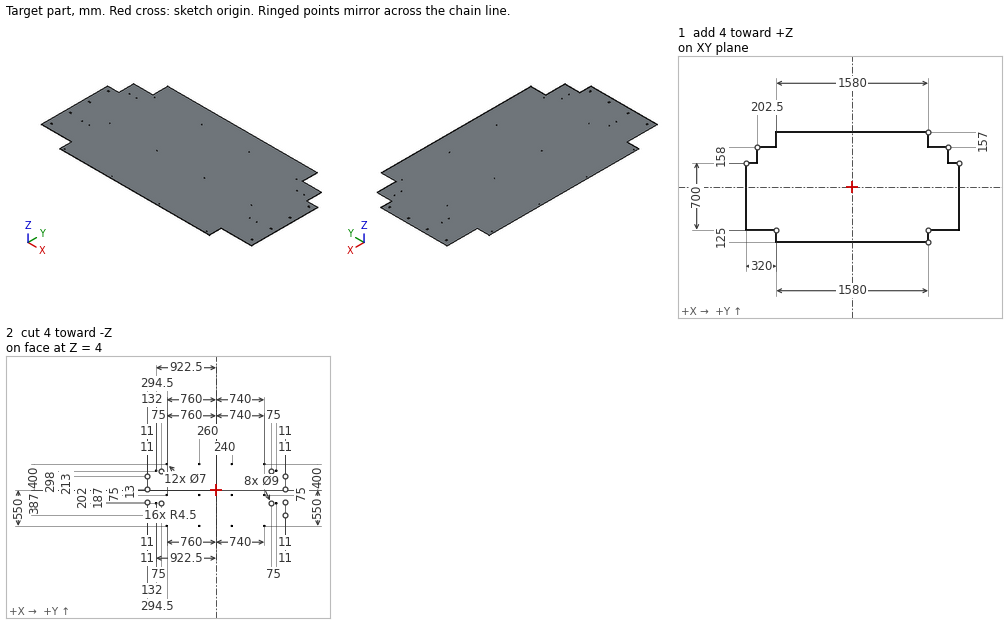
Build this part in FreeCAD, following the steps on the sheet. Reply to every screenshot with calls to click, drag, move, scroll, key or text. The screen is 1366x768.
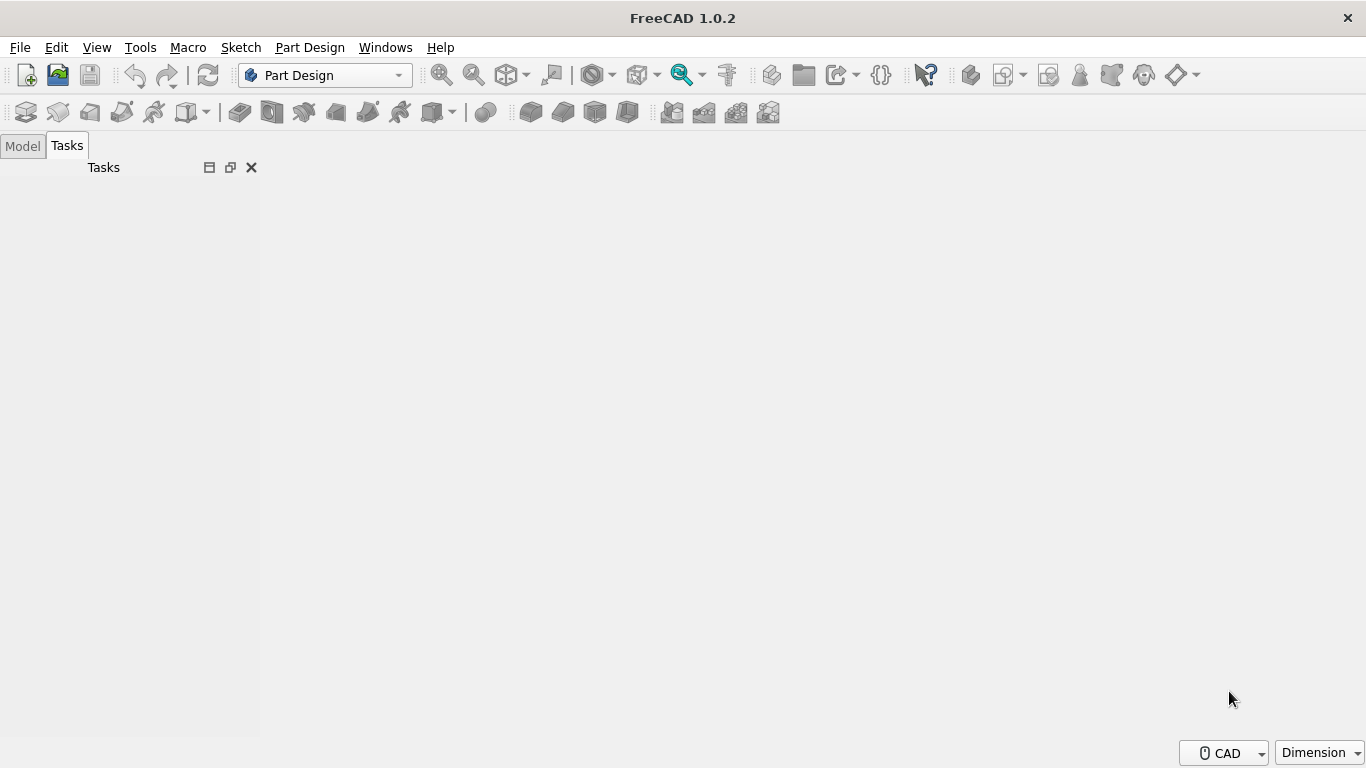
click(26, 76)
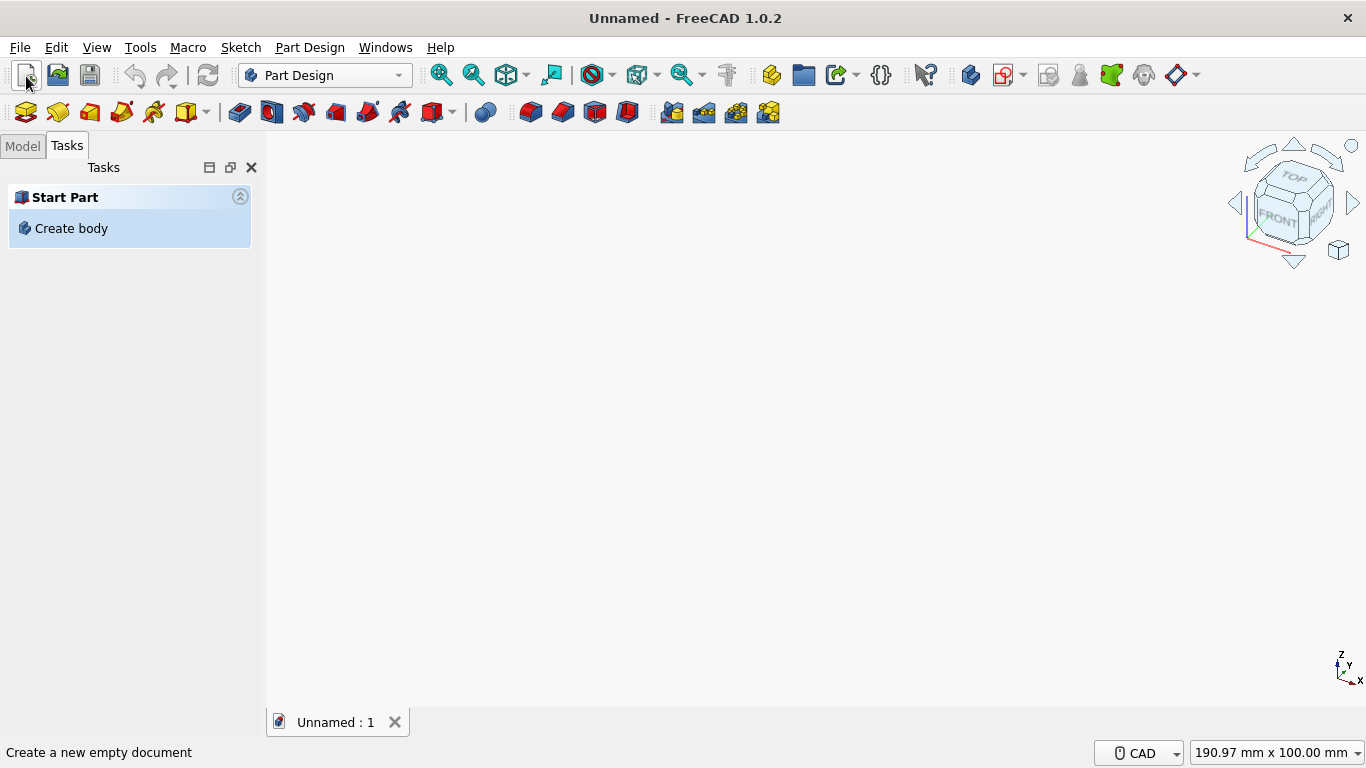
click(1004, 76)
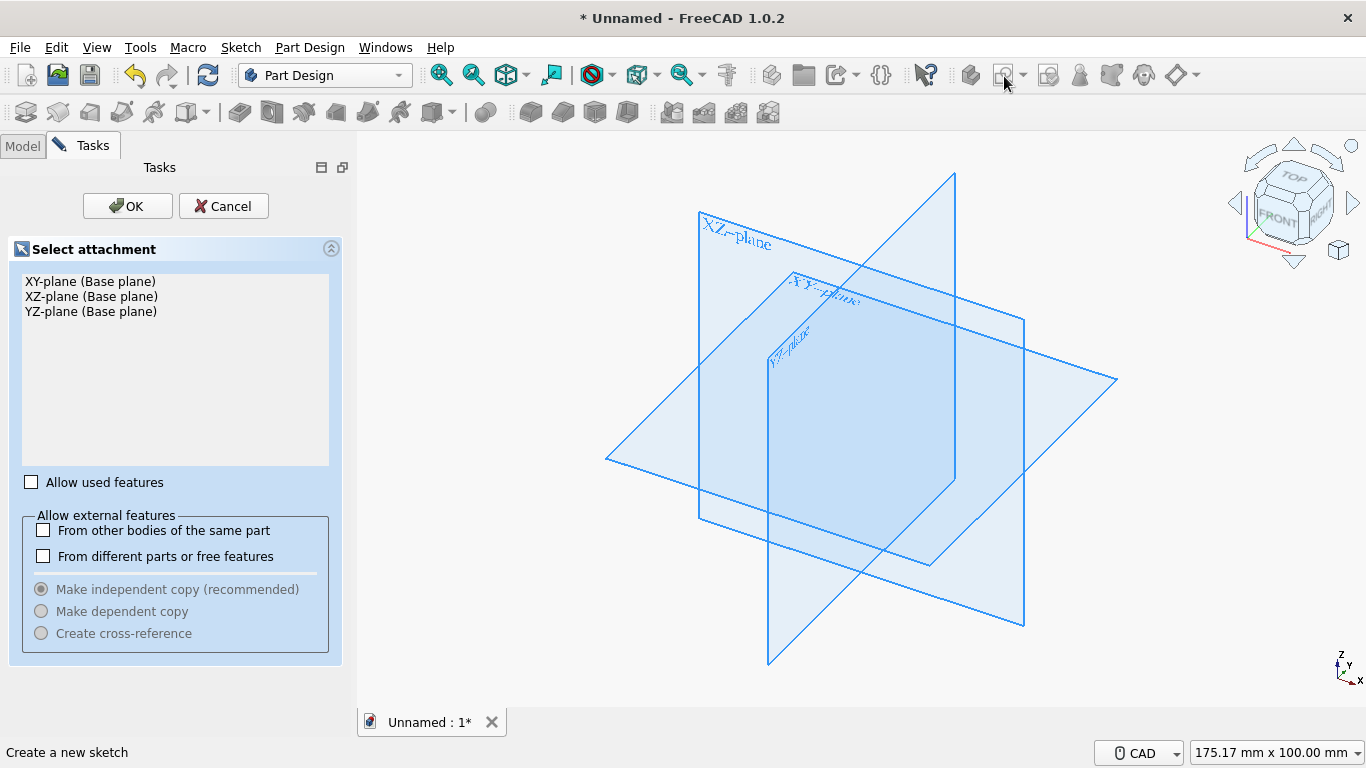
click(82, 282)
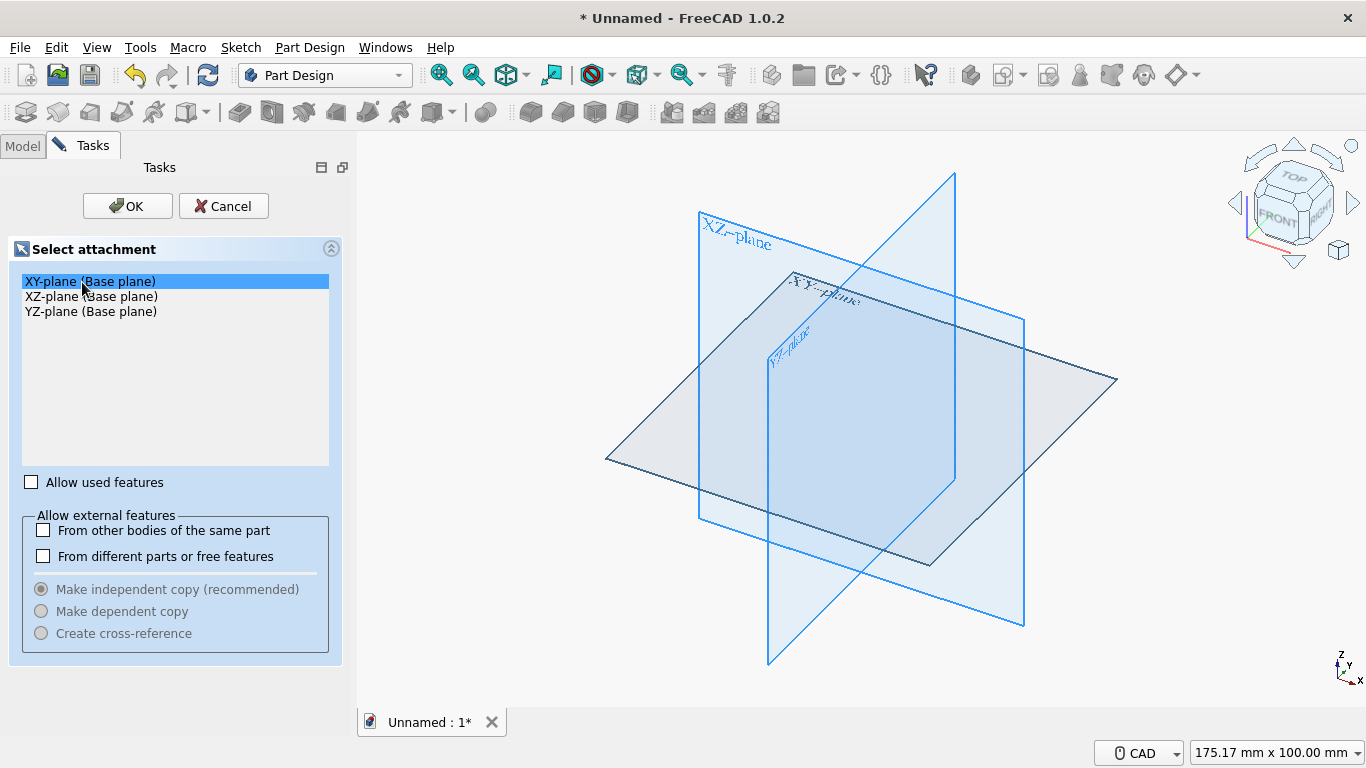
click(128, 206)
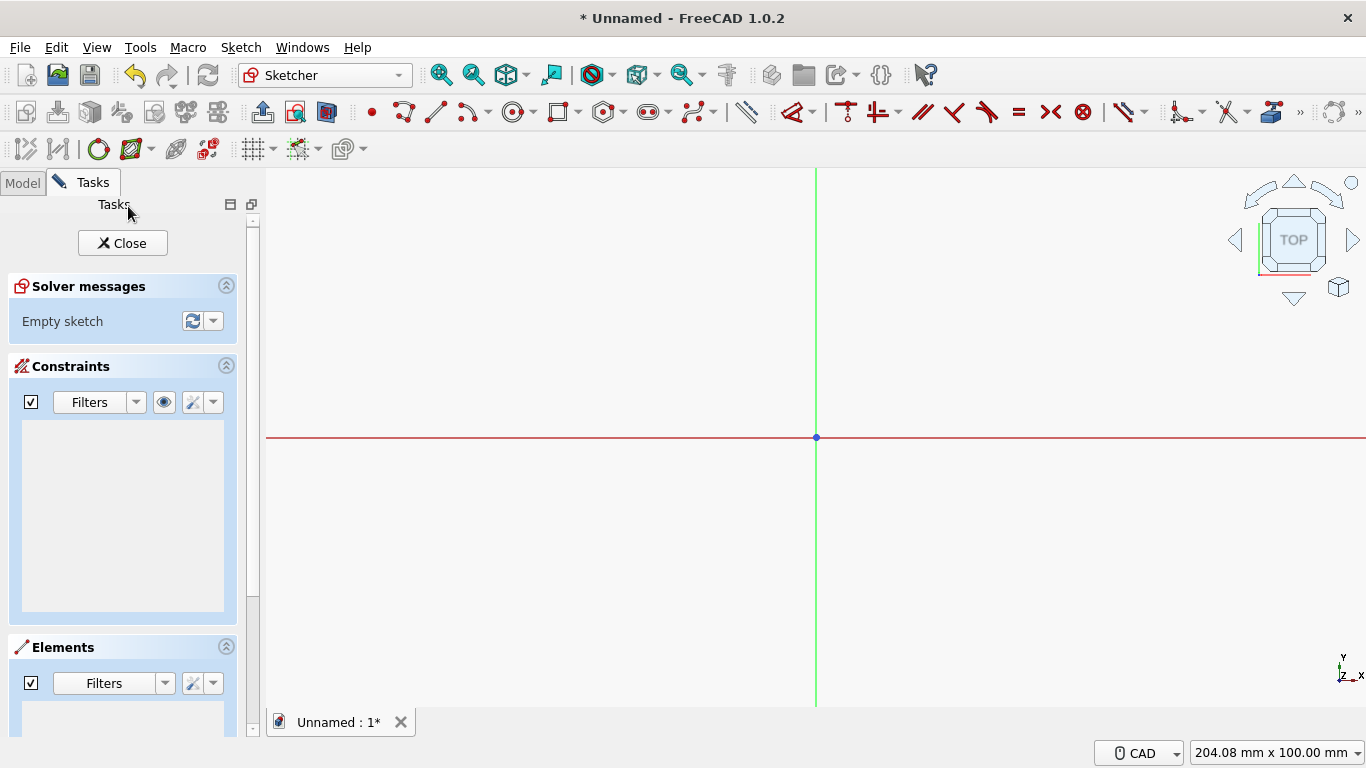
scroll(744, 438, down, 15)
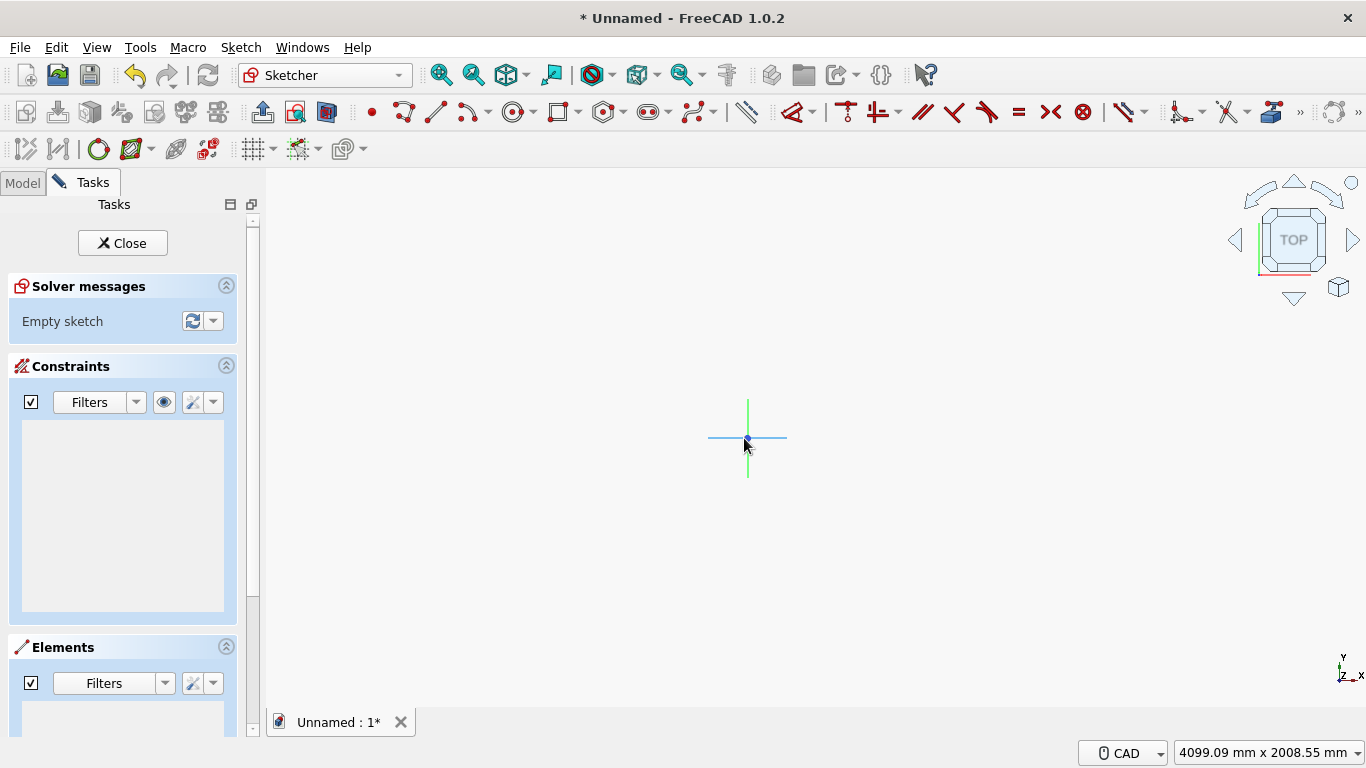
click(404, 112)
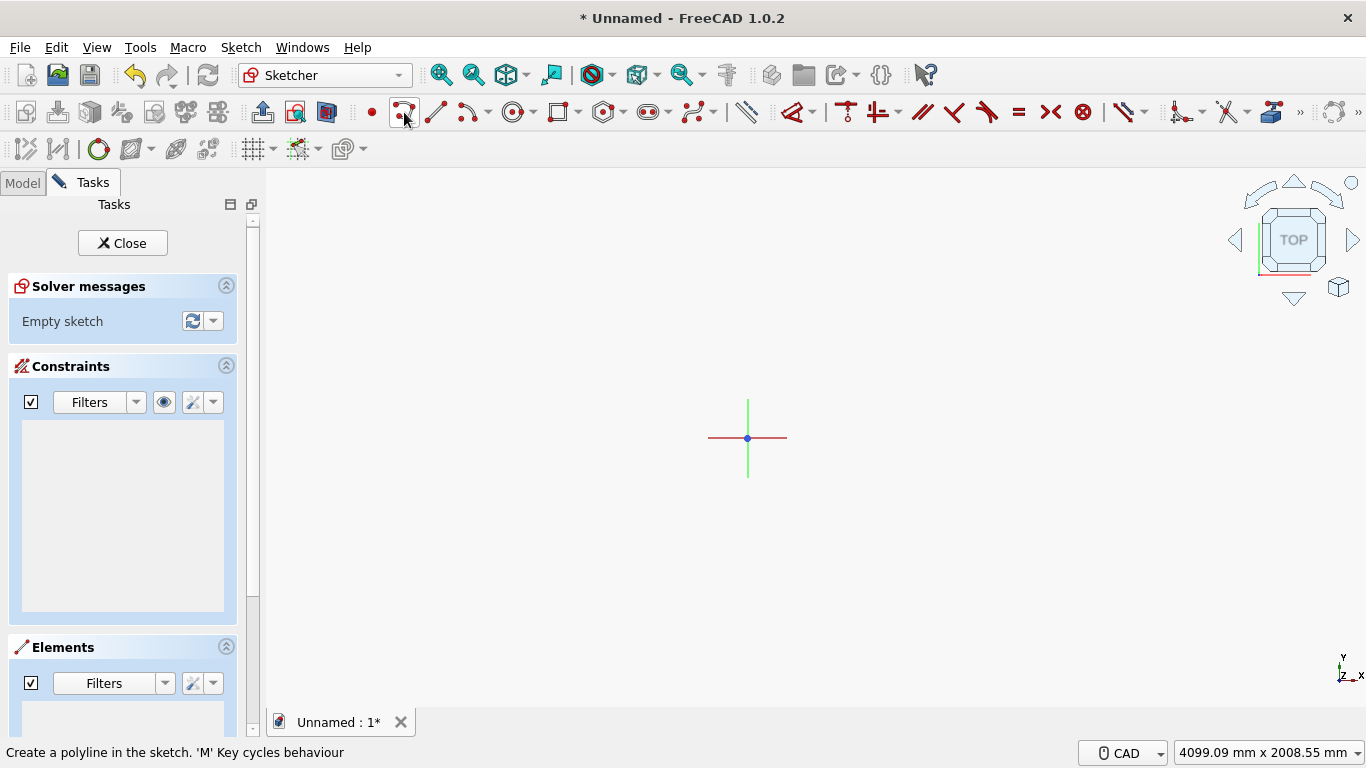
click(536, 328)
click(482, 328)
click(482, 370)
click(450, 370)
click(450, 558)
click(536, 558)
click(536, 591)
click(960, 591)
click(960, 558)
click(1046, 558)
click(1046, 370)
click(1014, 370)
click(1014, 328)
click(960, 328)
click(960, 285)
click(536, 285)
click(536, 329)
key(Escape)
key(Escape)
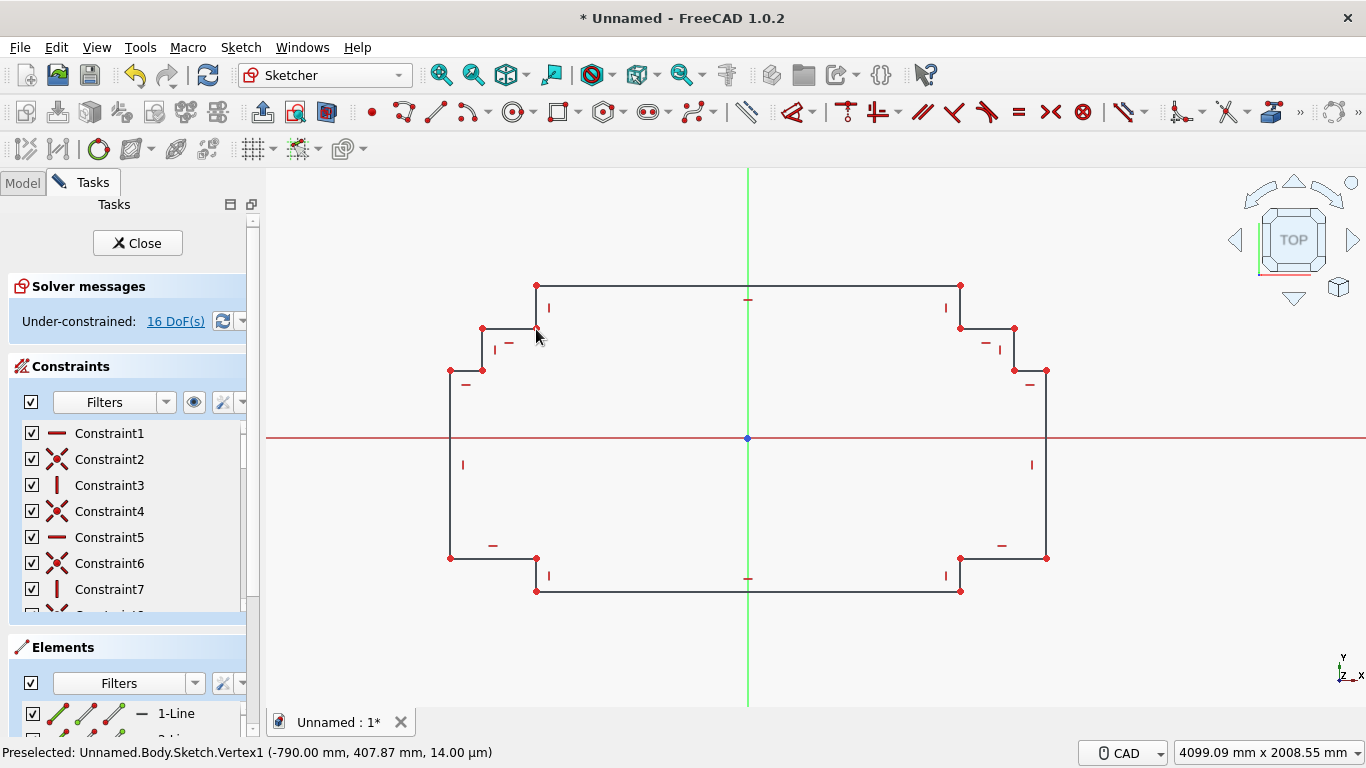
click(536, 559)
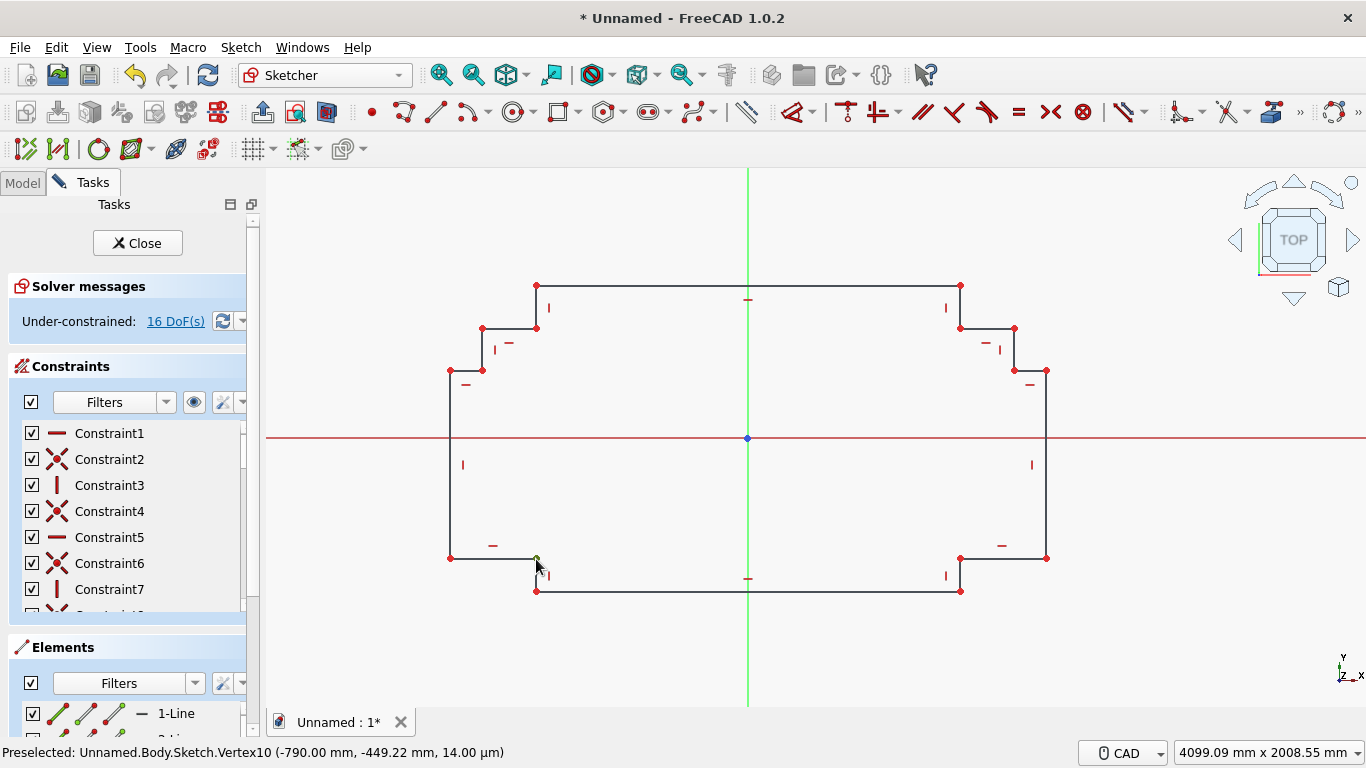
click(960, 559)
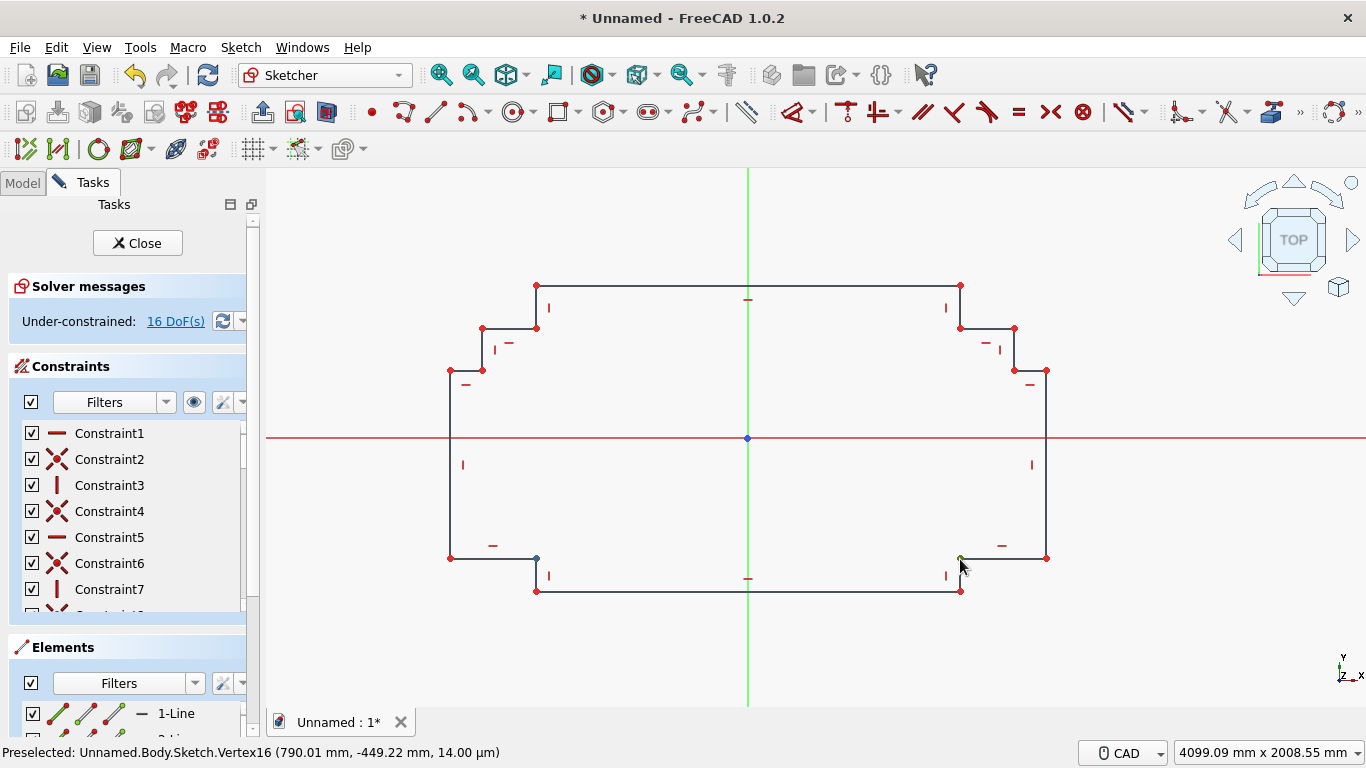
click(748, 644)